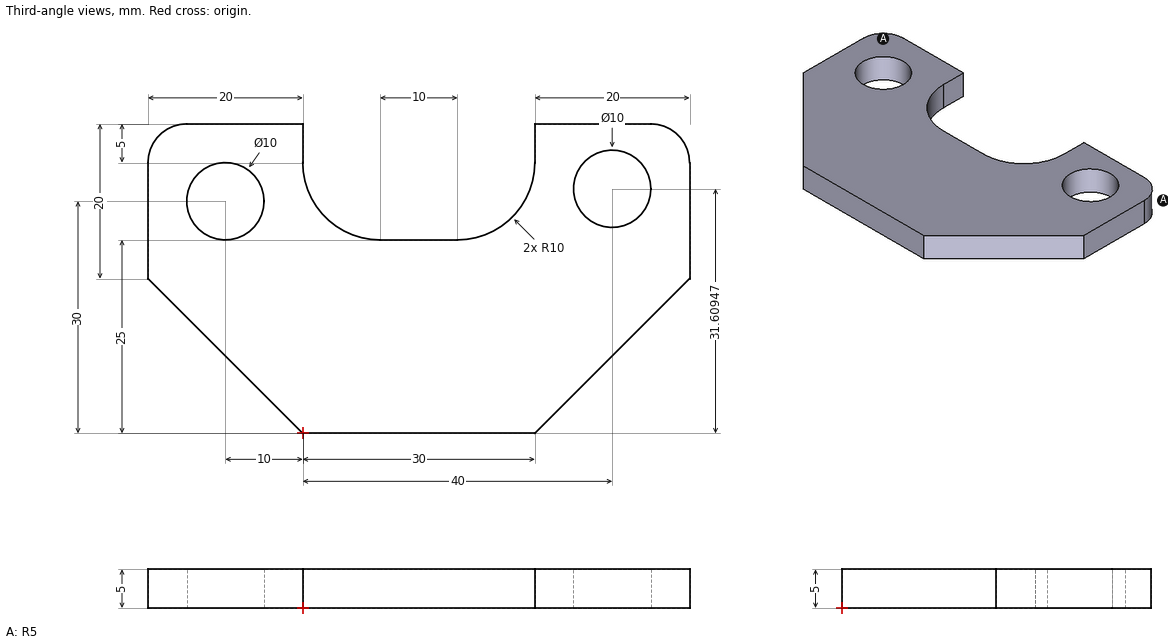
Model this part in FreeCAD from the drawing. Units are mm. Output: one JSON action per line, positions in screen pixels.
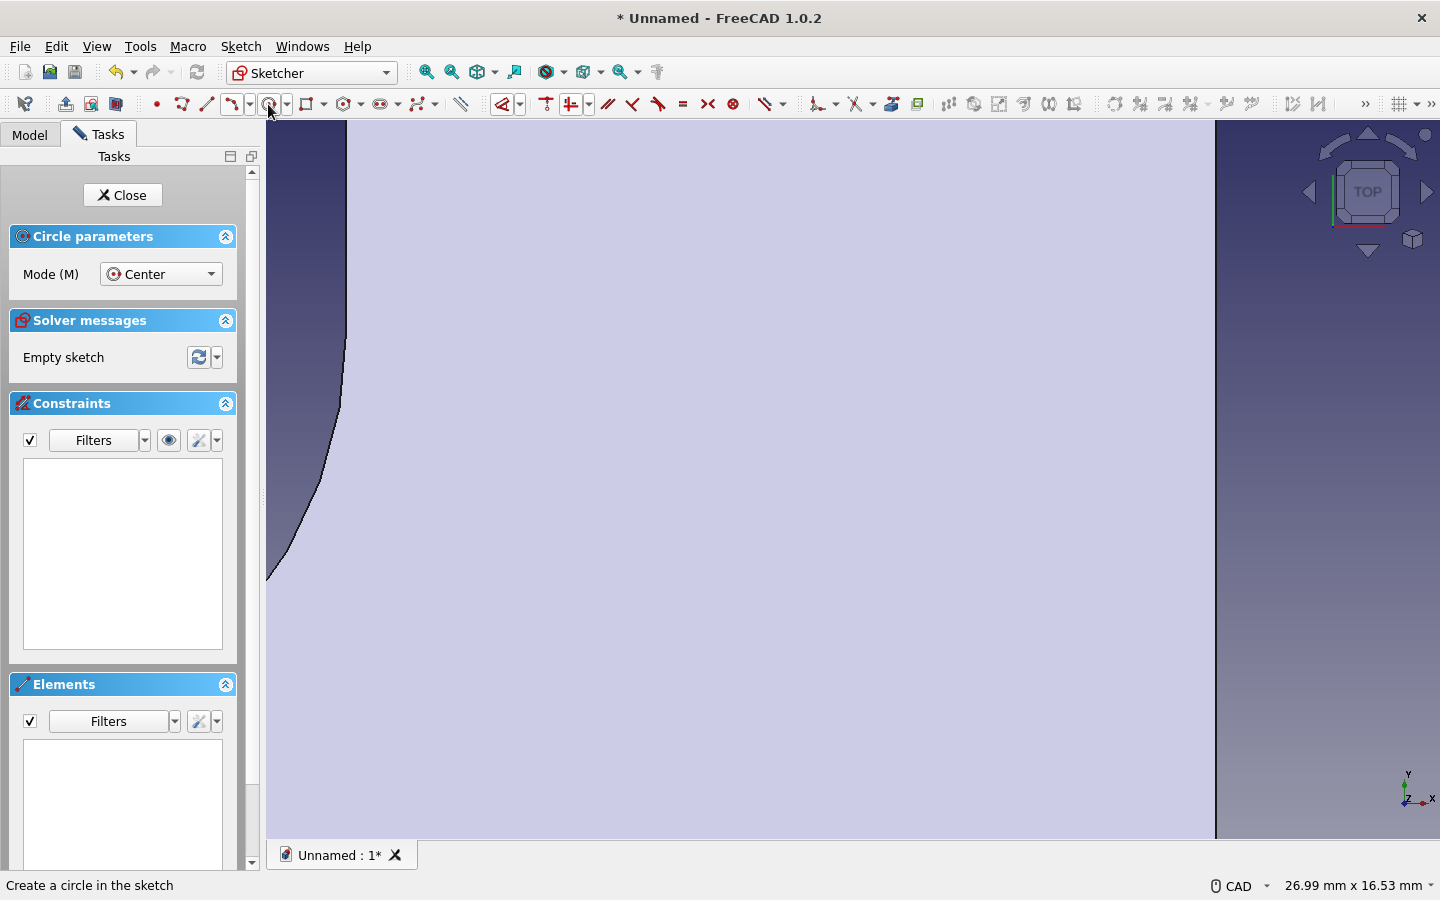
{"action": "left_click", "coordinate": [781, 480]}
{"action": "left_click", "coordinate": [935, 326]}
{"action": "key", "text": "Escape"}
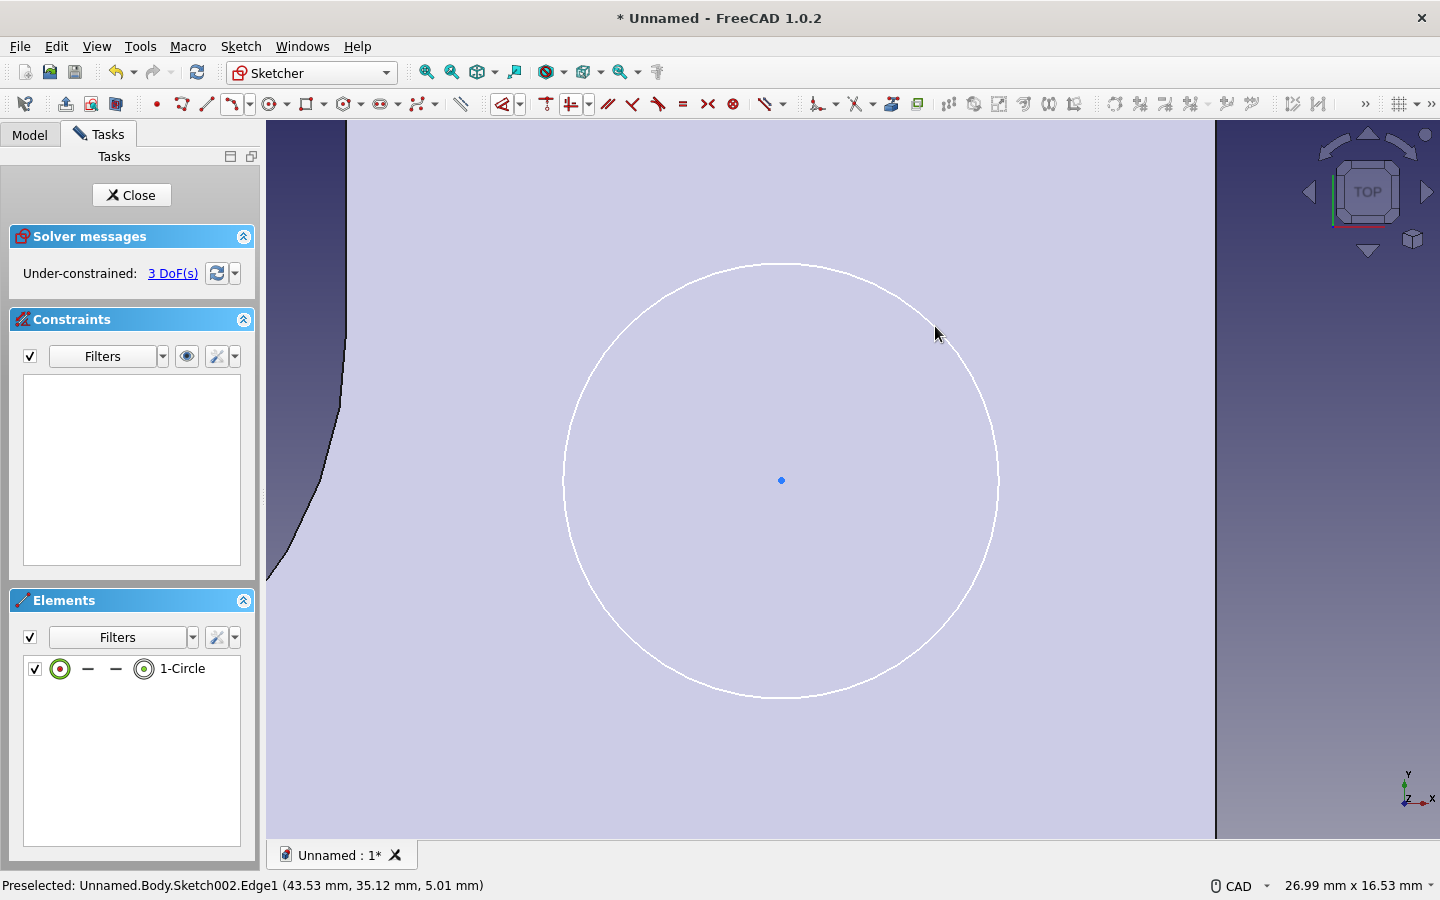
{"action": "left_click", "coordinate": [935, 327]}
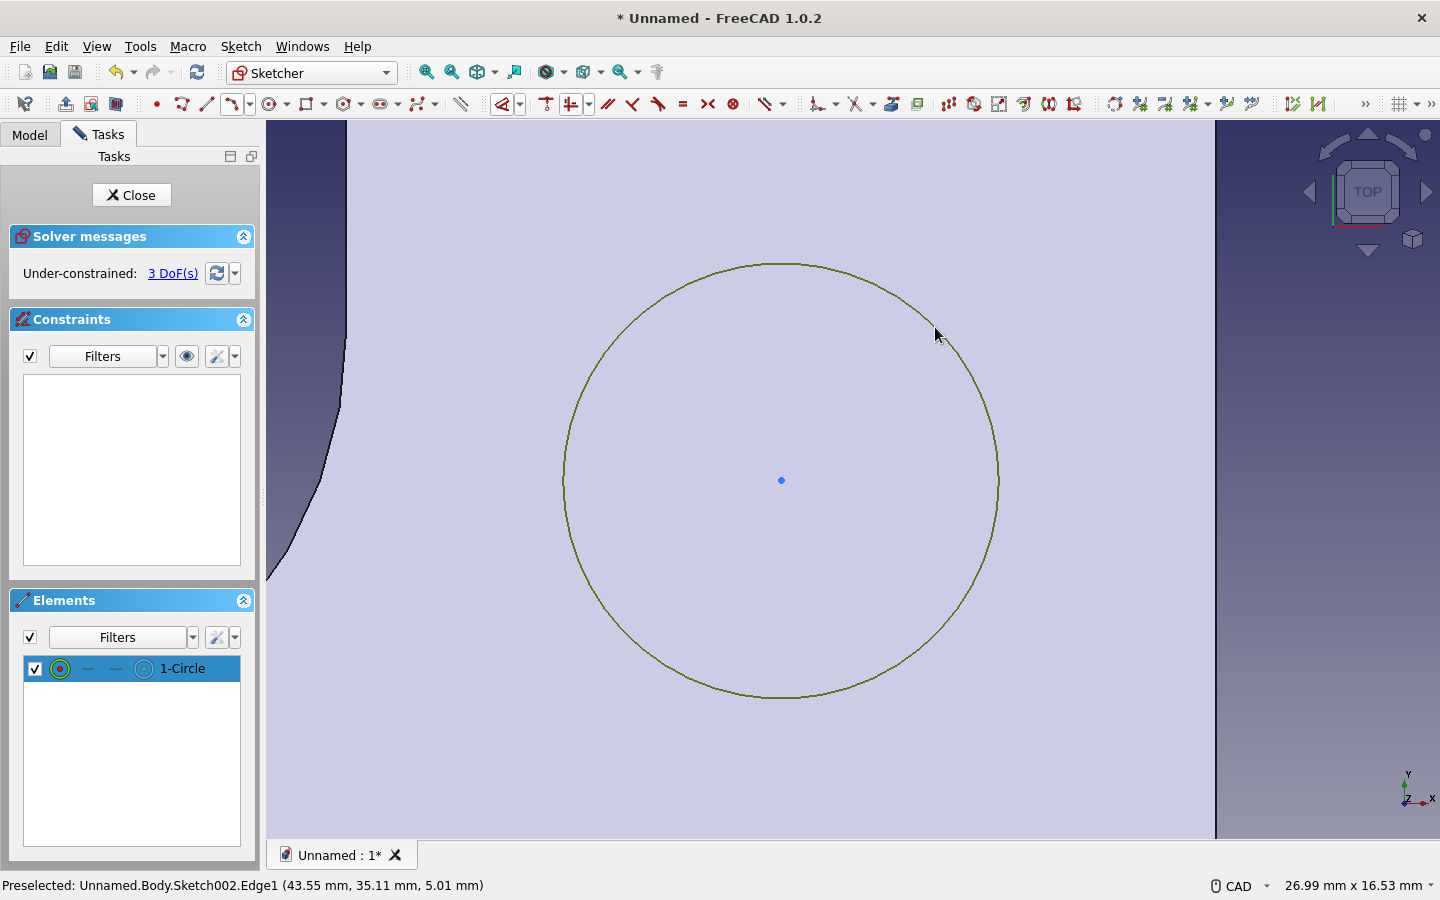
{"action": "left_click", "coordinate": [520, 104]}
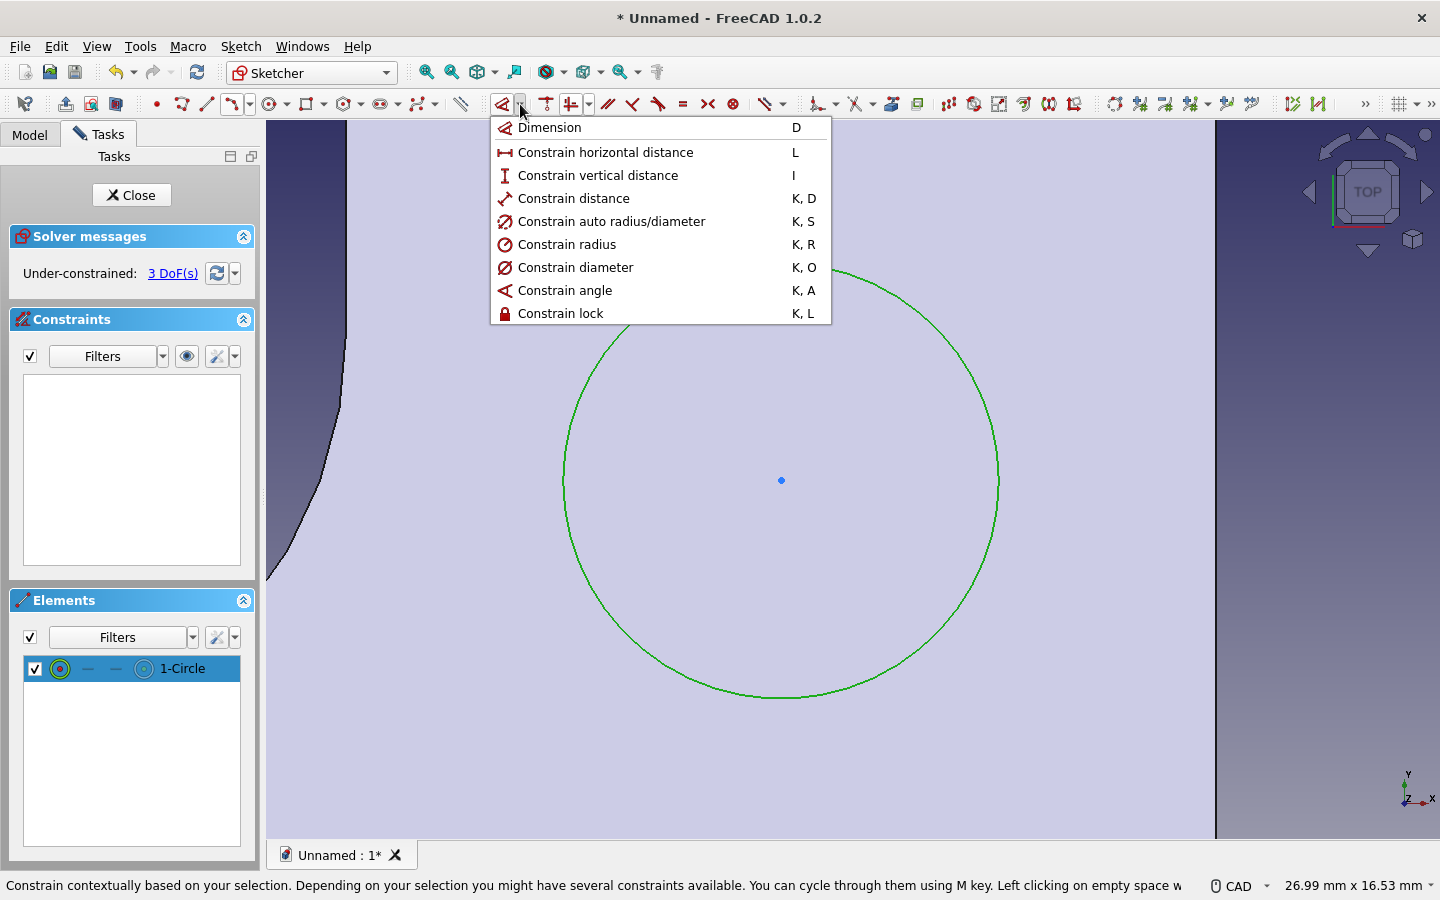
{"action": "left_click", "coordinate": [661, 268]}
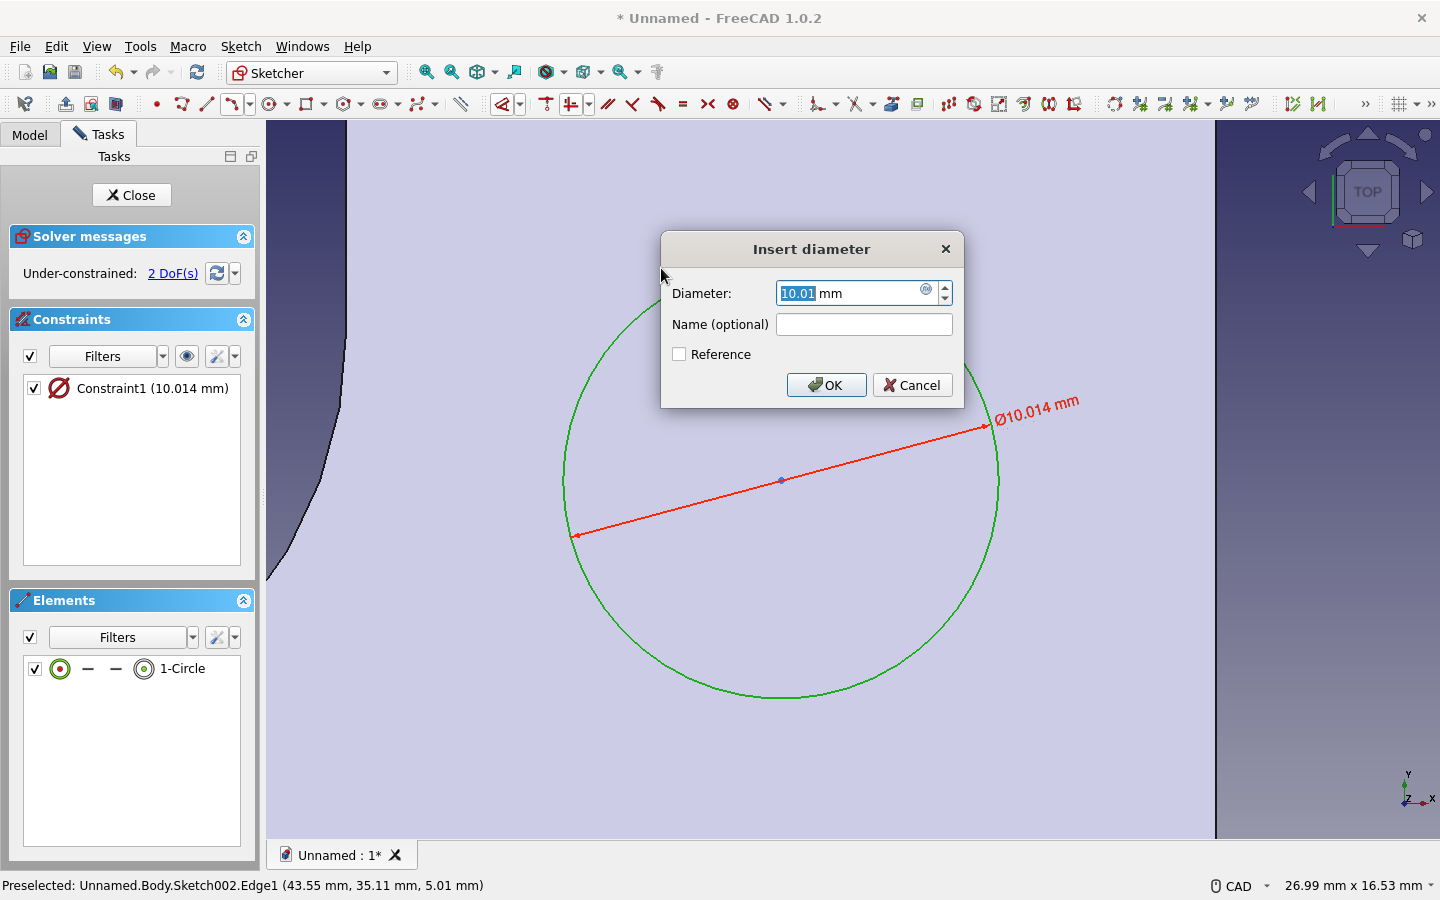
{"action": "type", "text": "10"}
{"action": "key", "text": "Return"}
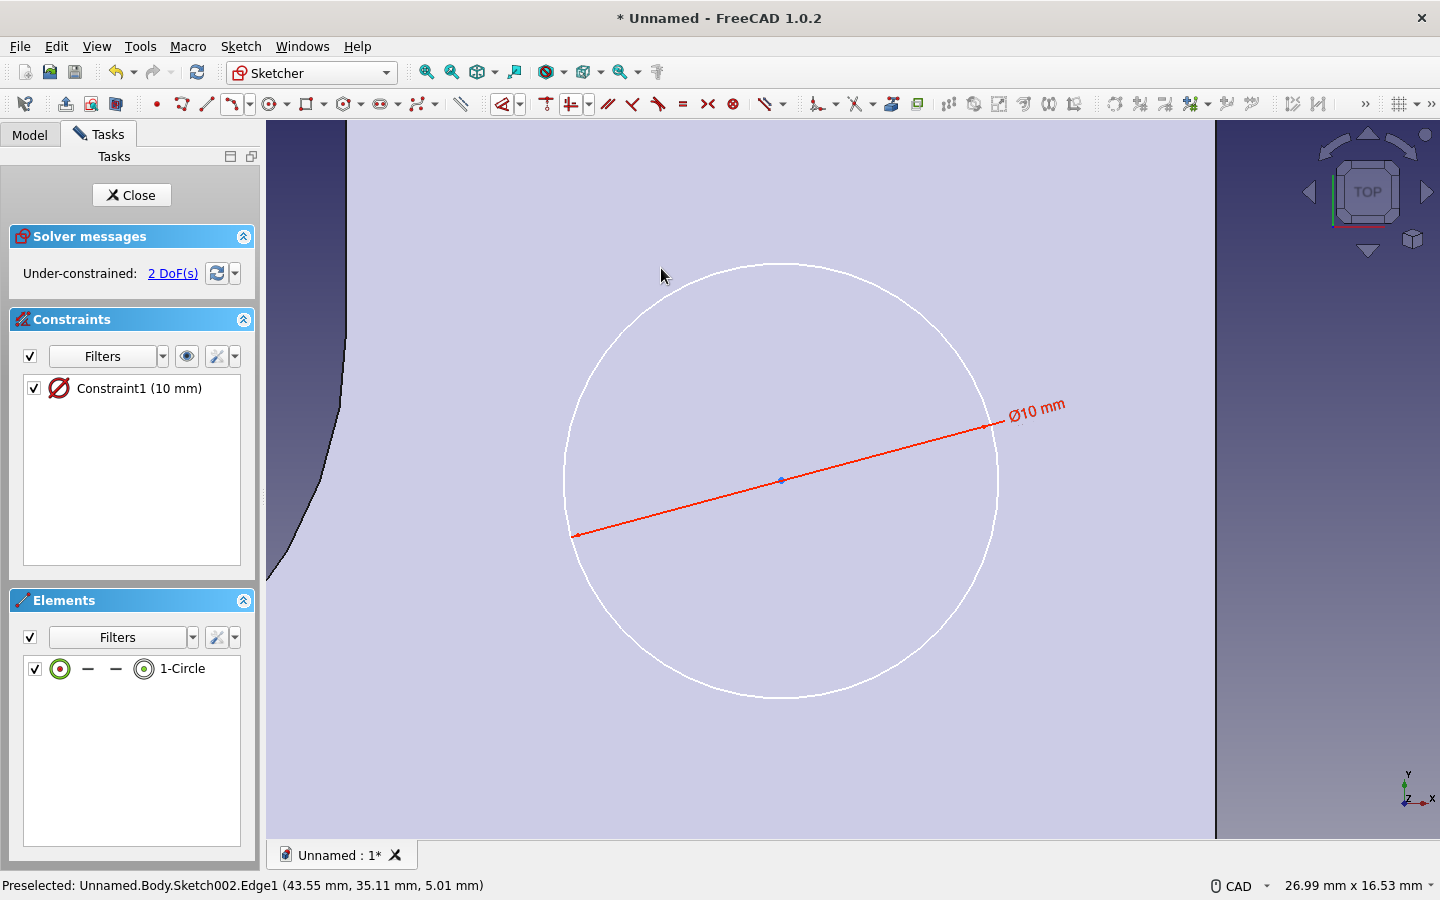
{"action": "left_click", "coordinate": [781, 481]}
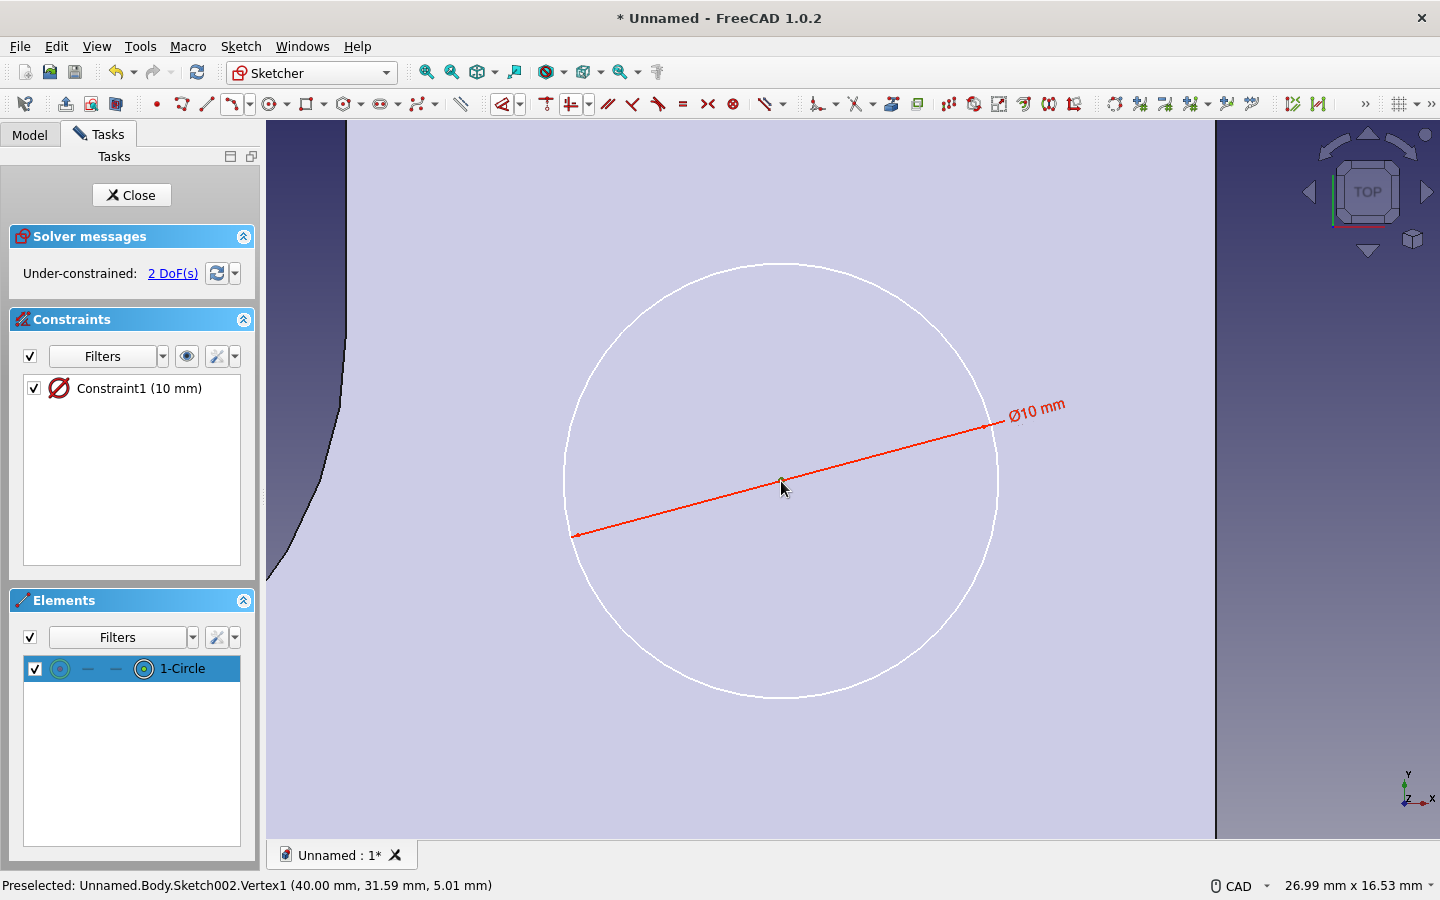
{"action": "left_click", "coordinate": [520, 104]}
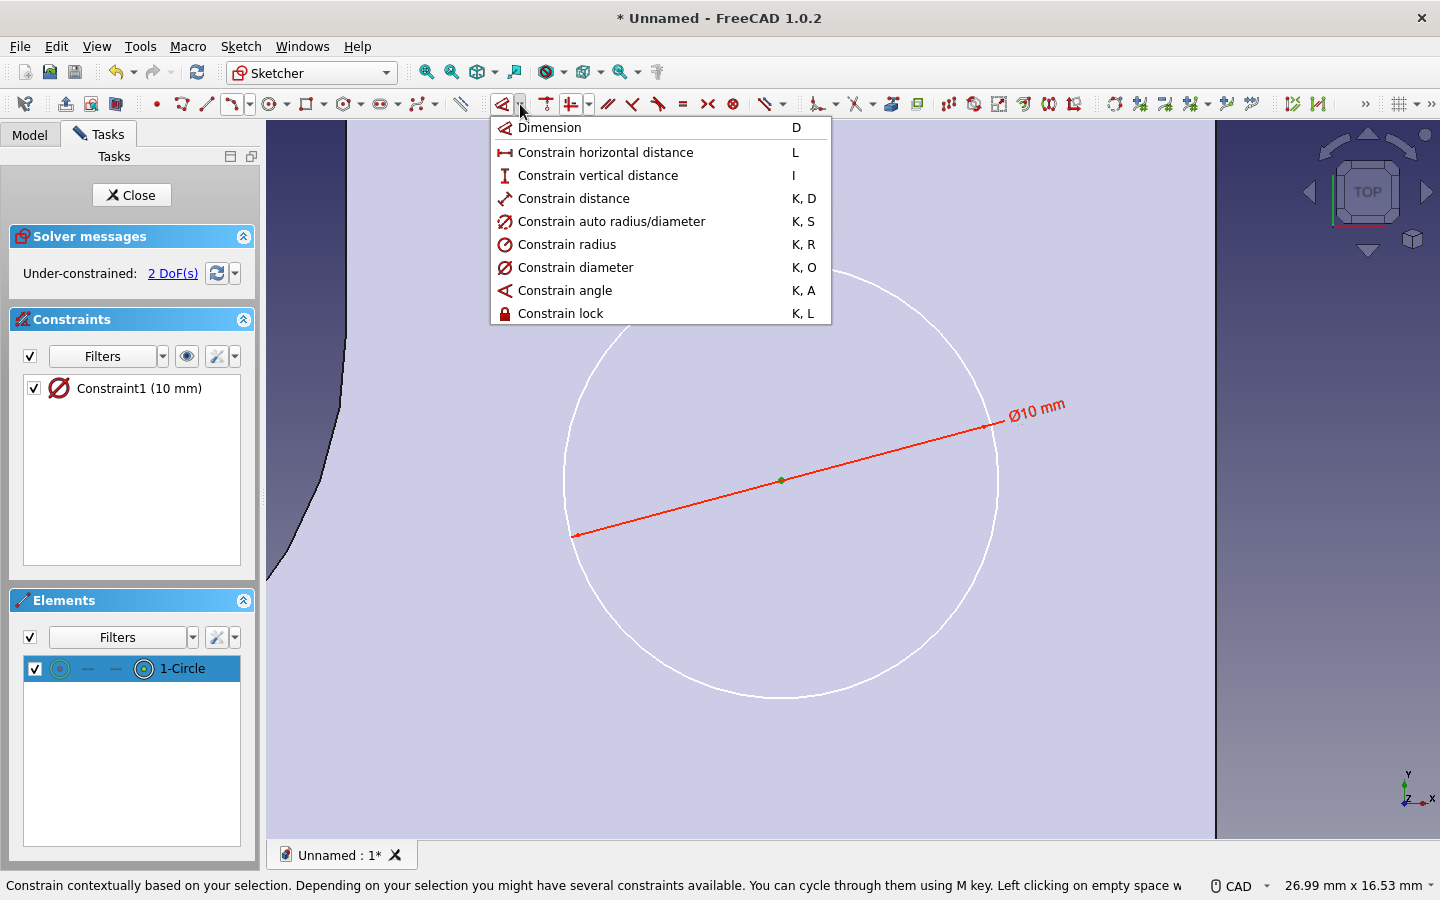
{"action": "left_click", "coordinate": [661, 152]}